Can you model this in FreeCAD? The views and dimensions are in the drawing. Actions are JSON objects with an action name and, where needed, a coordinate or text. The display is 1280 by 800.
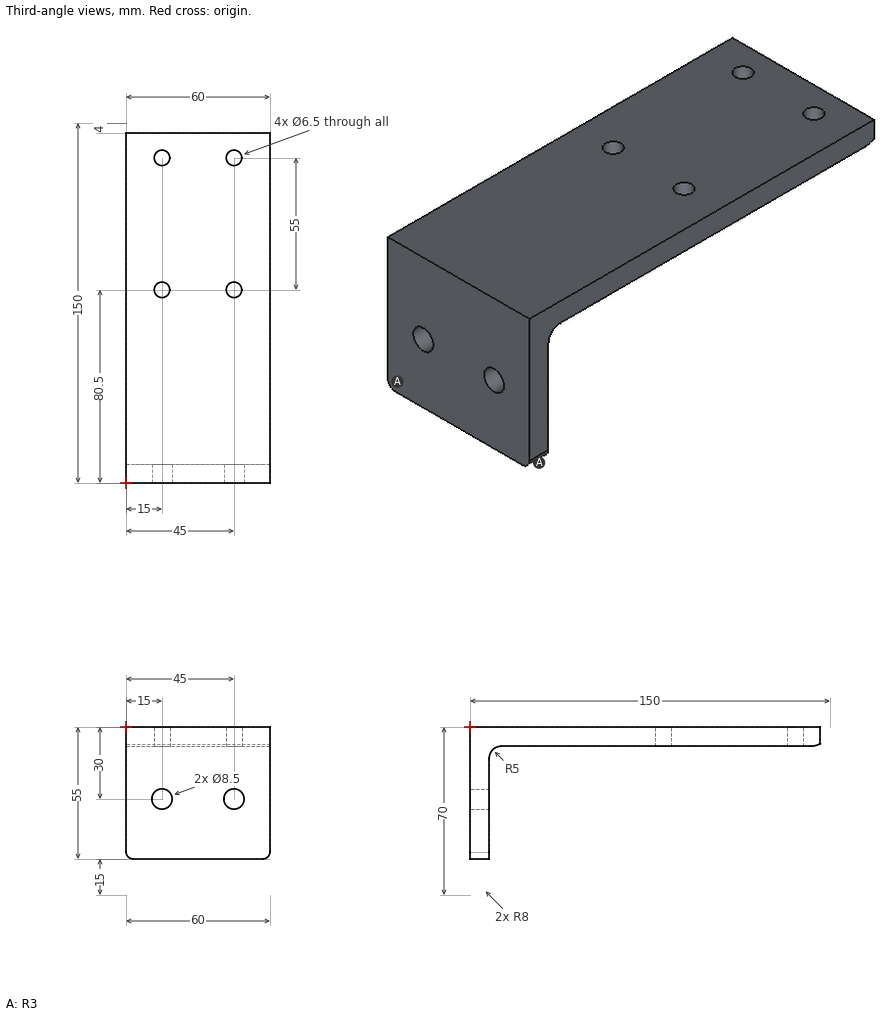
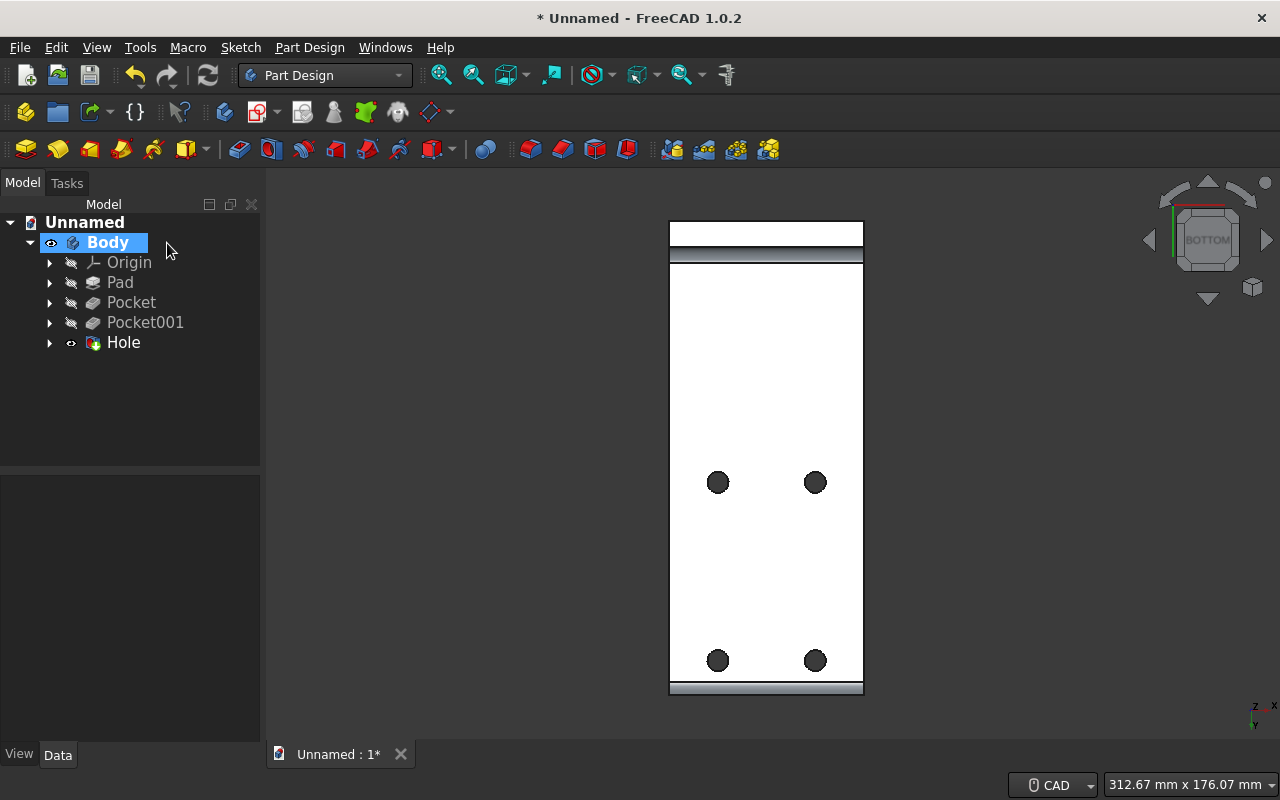
{"action": "left_click", "coordinate": [669, 233]}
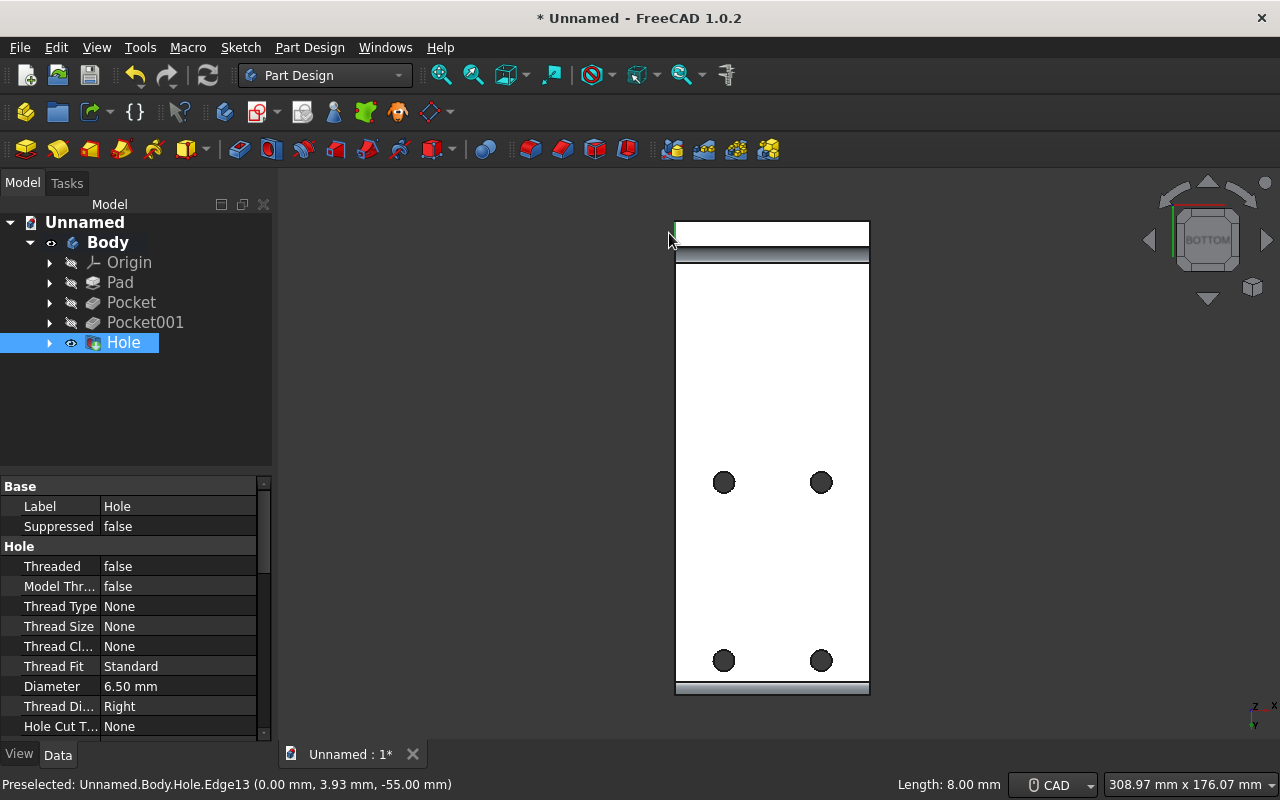
{"action": "left_click", "coordinate": [870, 233], "text": "ctrl"}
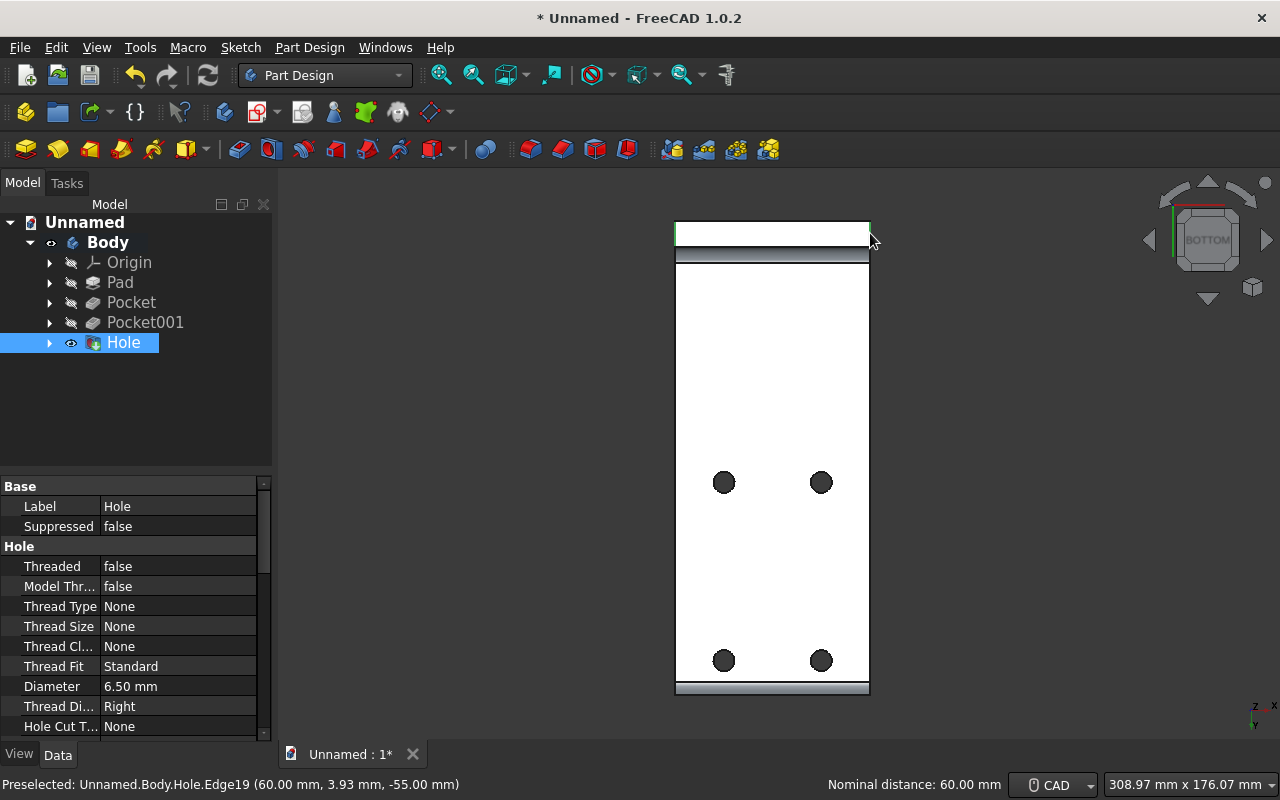
{"action": "left_click", "coordinate": [532, 150]}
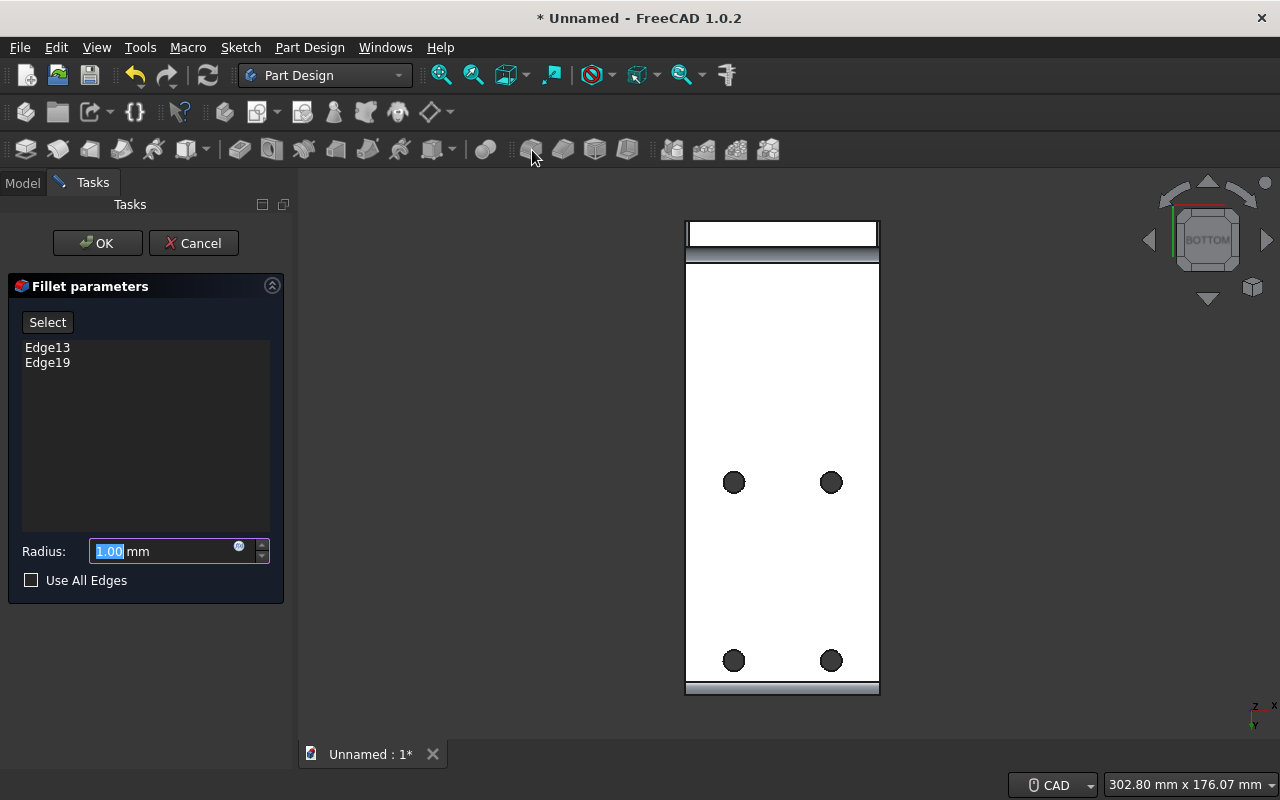
{"action": "type", "text": "3"}
{"action": "key", "text": "Tab"}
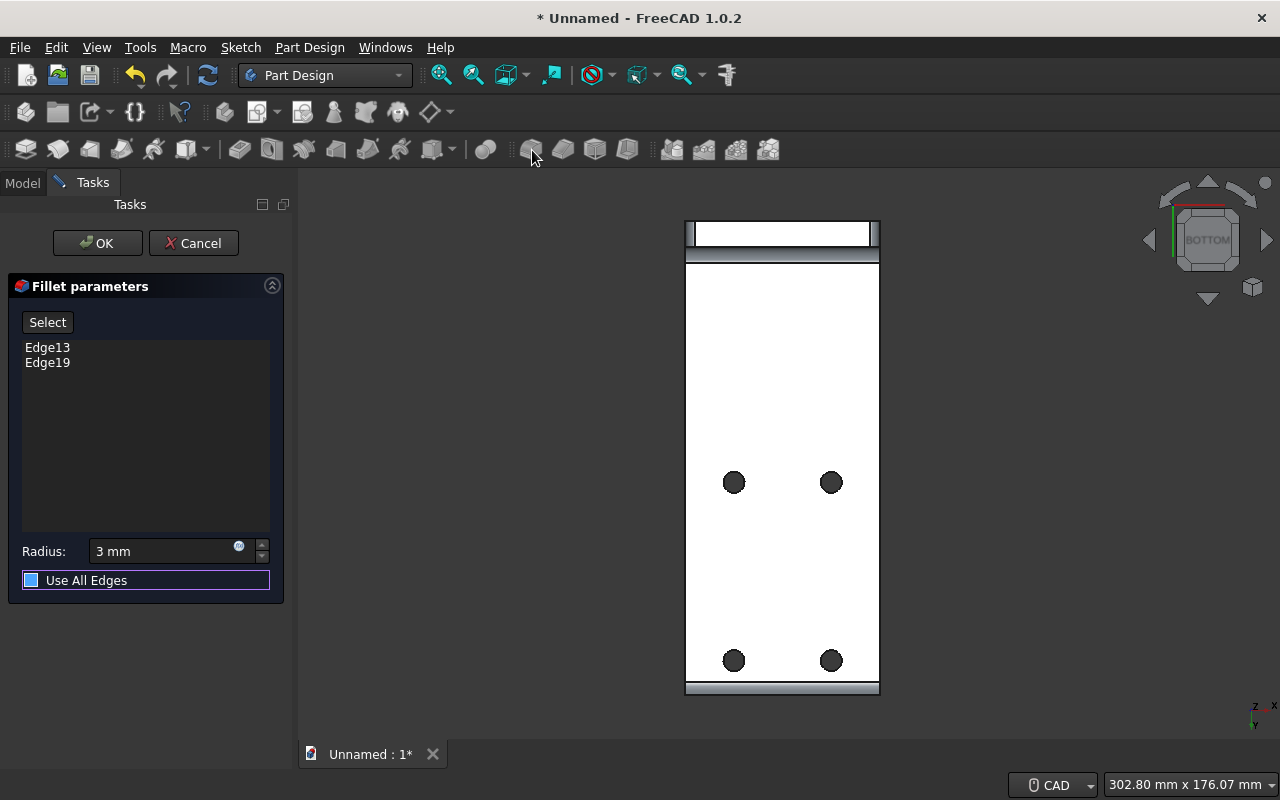
{"action": "left_click", "coordinate": [98, 243]}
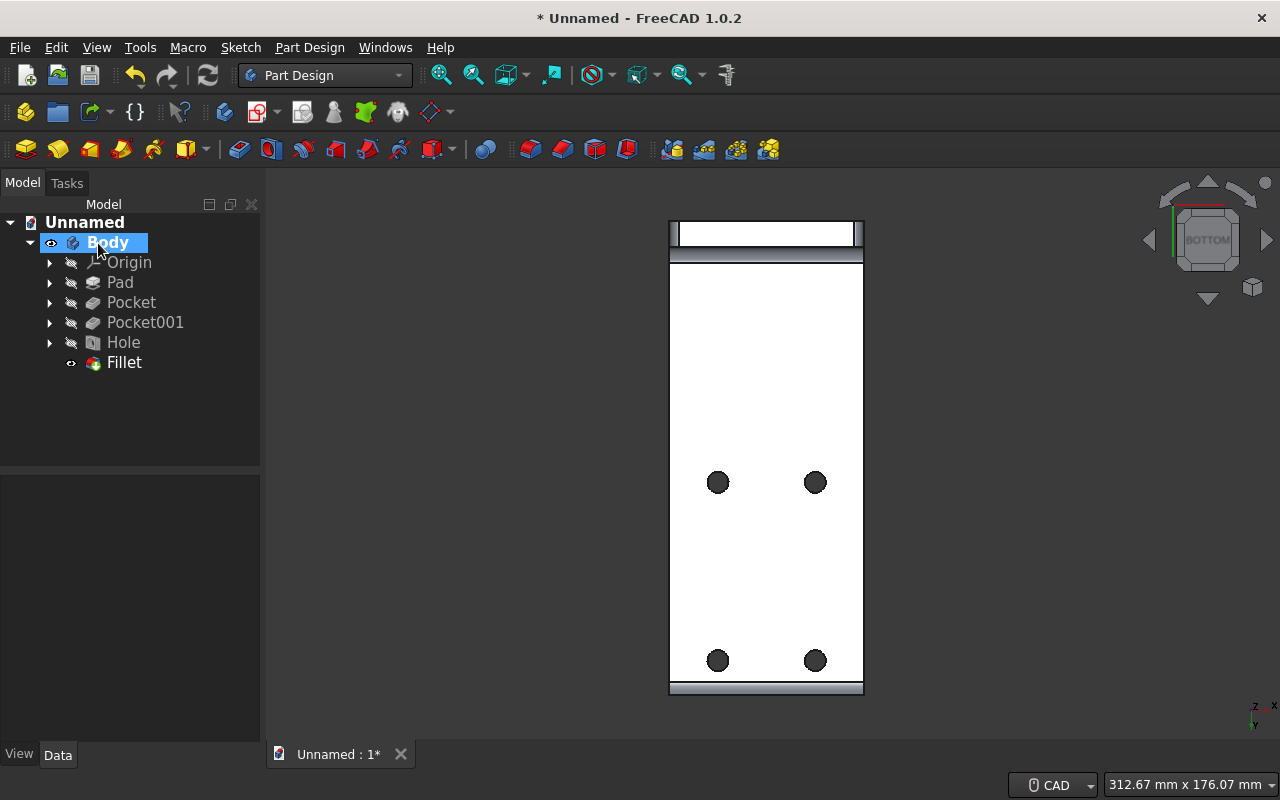
{"action": "key", "text": "4"}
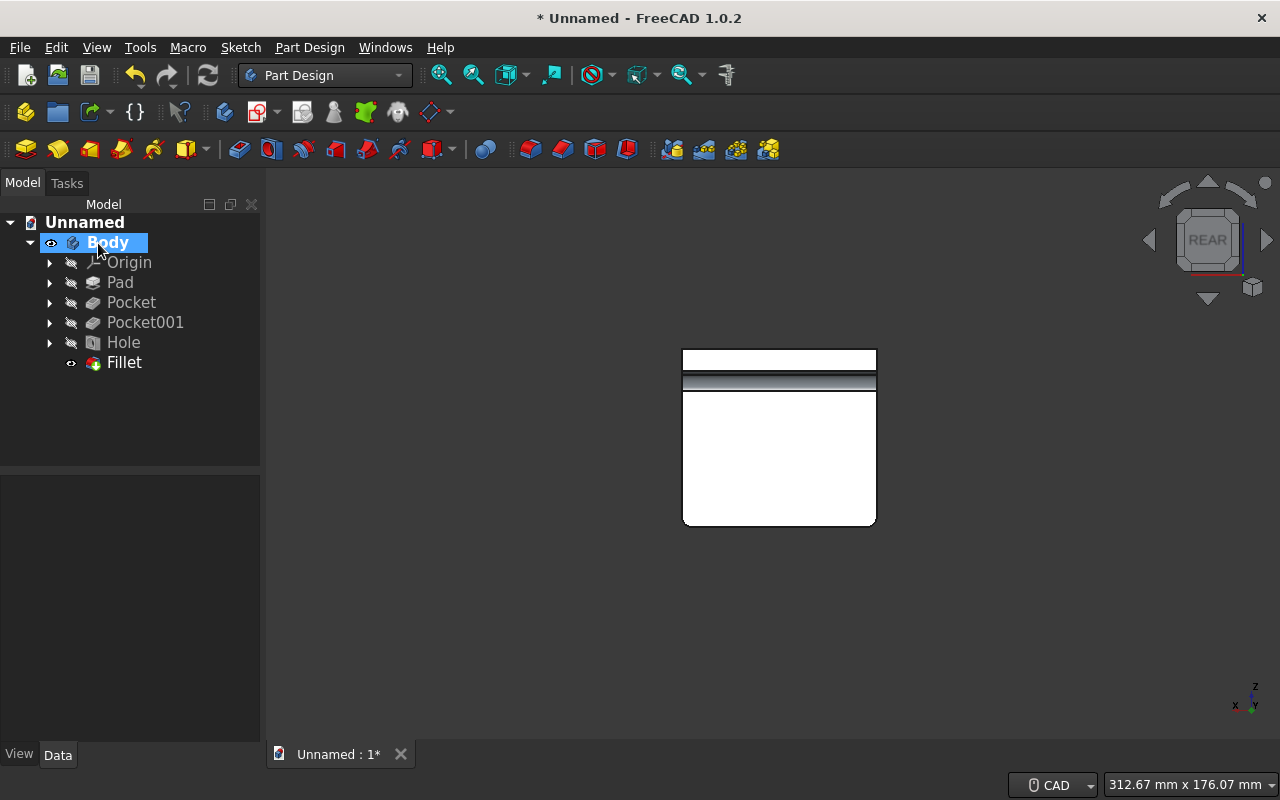
{"action": "left_click", "coordinate": [442, 76]}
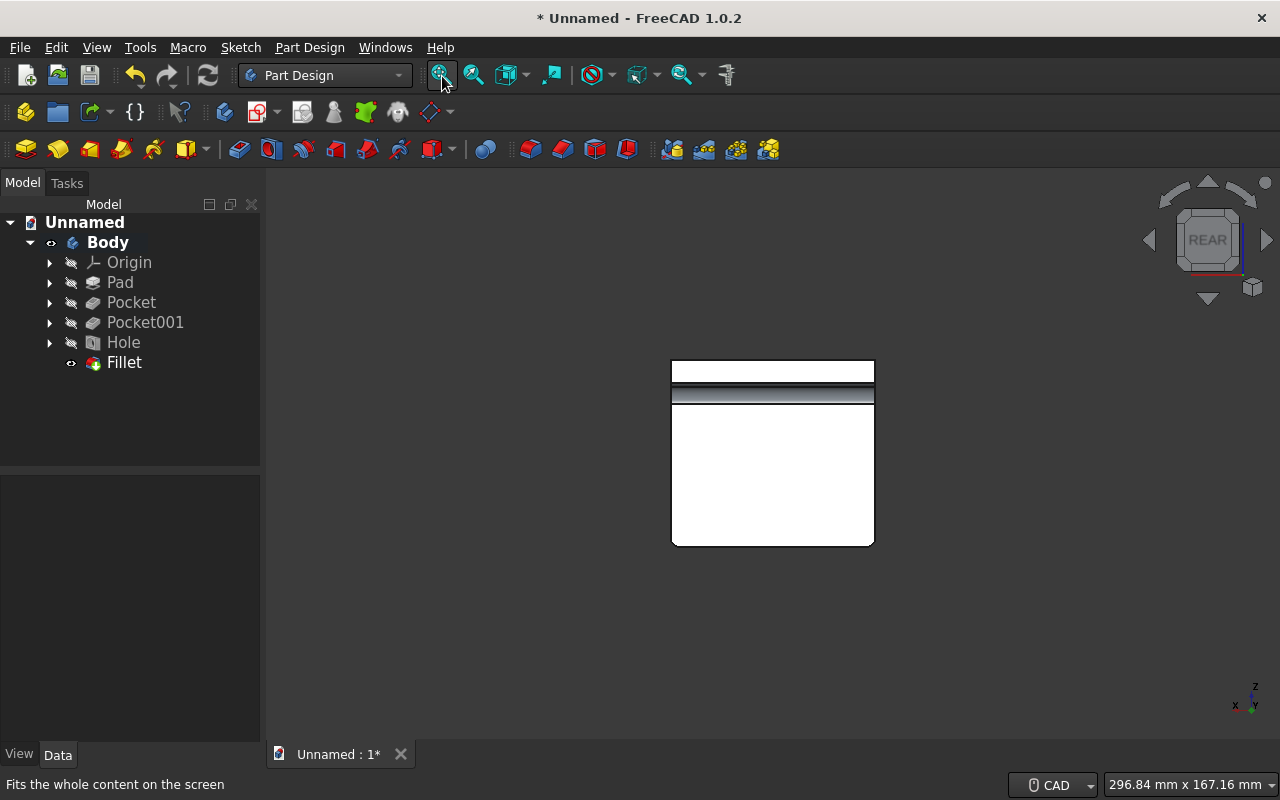
{"action": "left_click", "coordinate": [744, 475]}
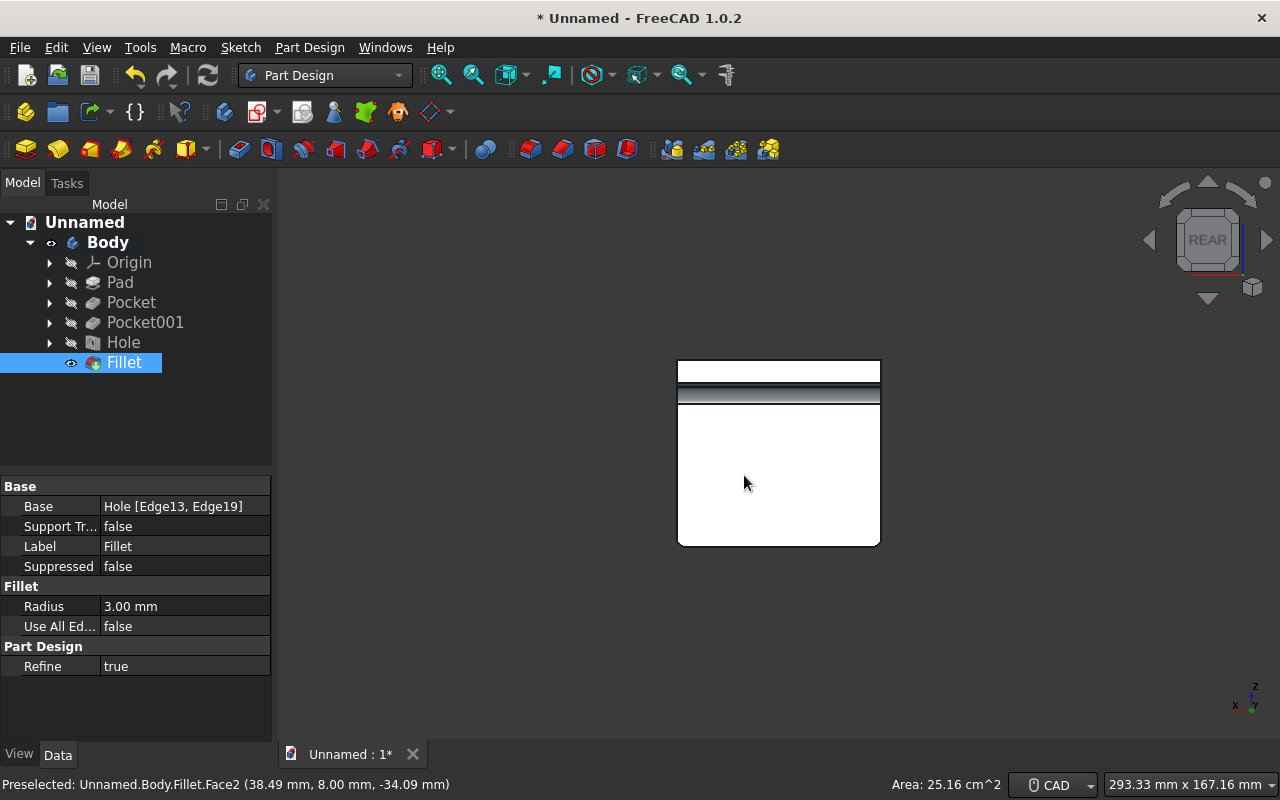
{"action": "left_click", "coordinate": [258, 112]}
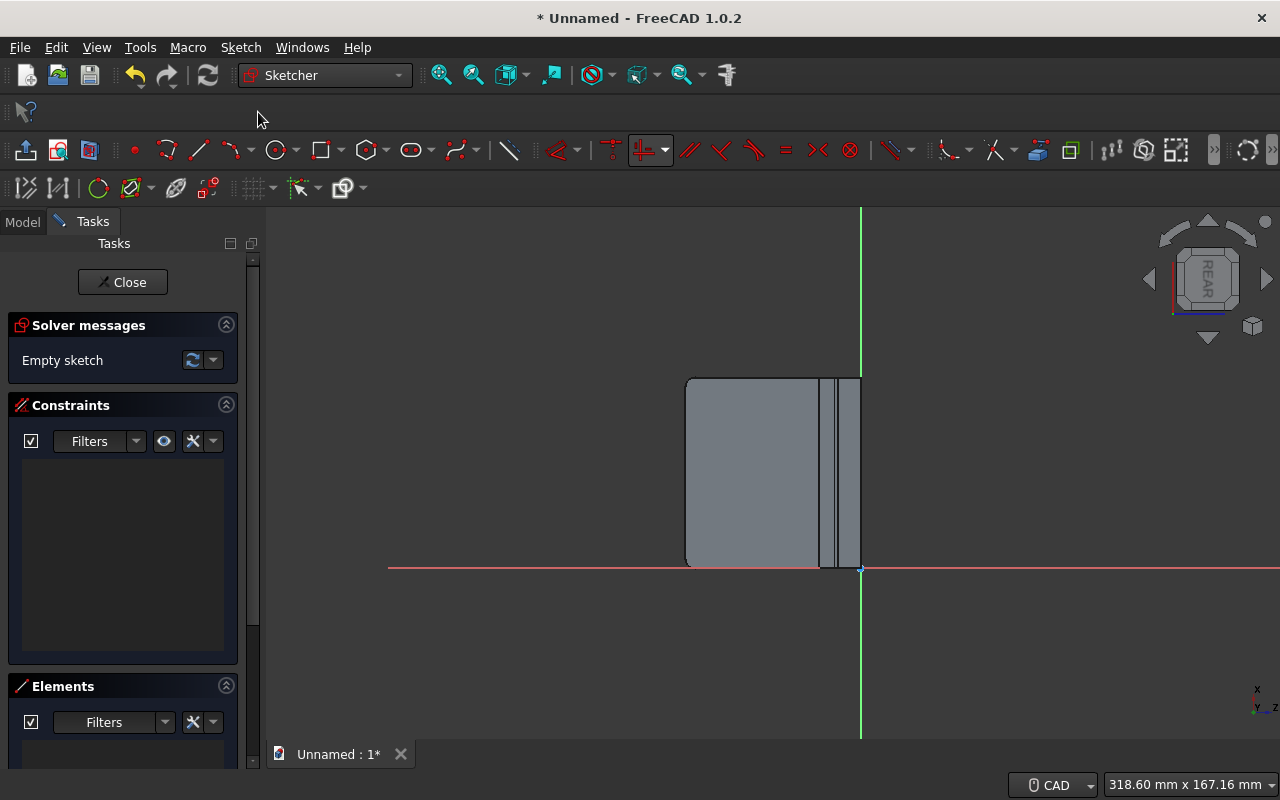
{"action": "scroll", "coordinate": [889, 504], "scroll_direction": "up", "scroll_amount": 4}